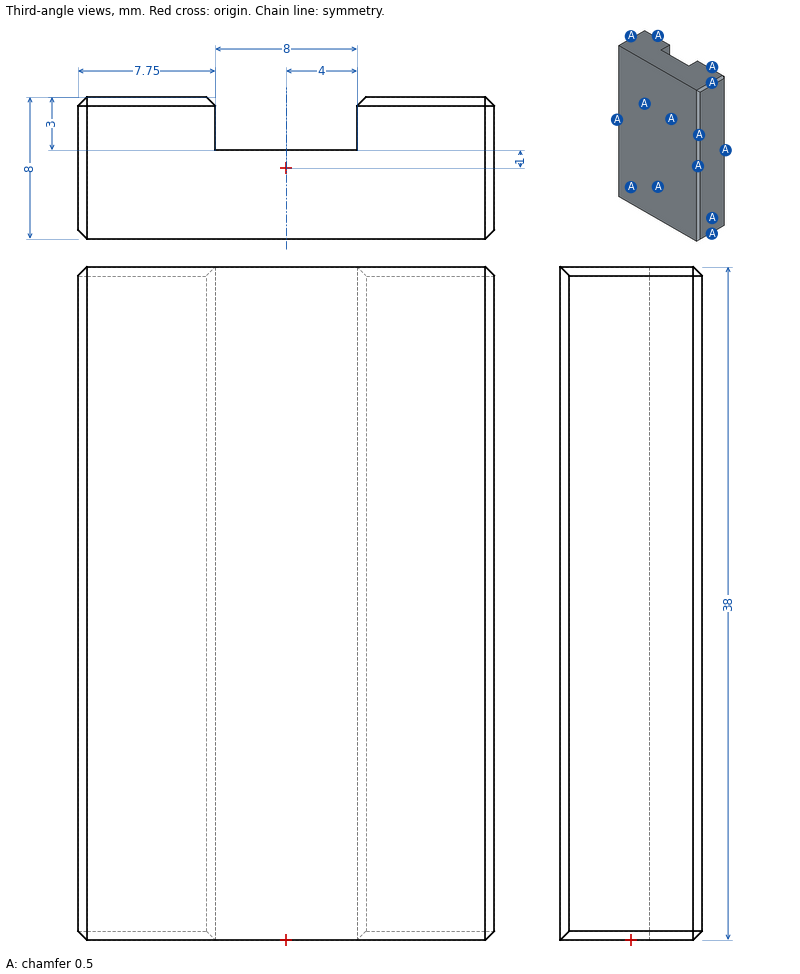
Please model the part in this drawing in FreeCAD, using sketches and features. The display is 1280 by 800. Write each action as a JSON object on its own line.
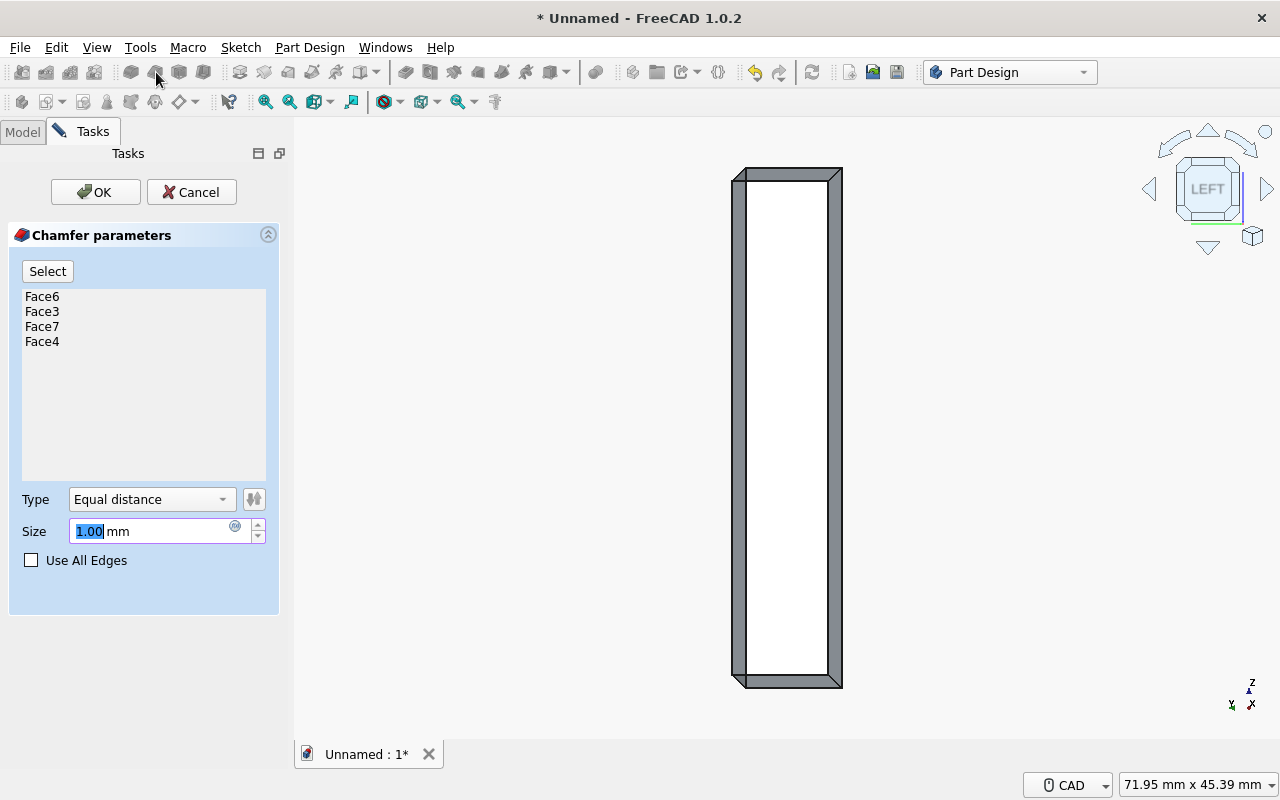
{"action": "type", "text": "0.5"}
{"action": "key", "text": "Tab"}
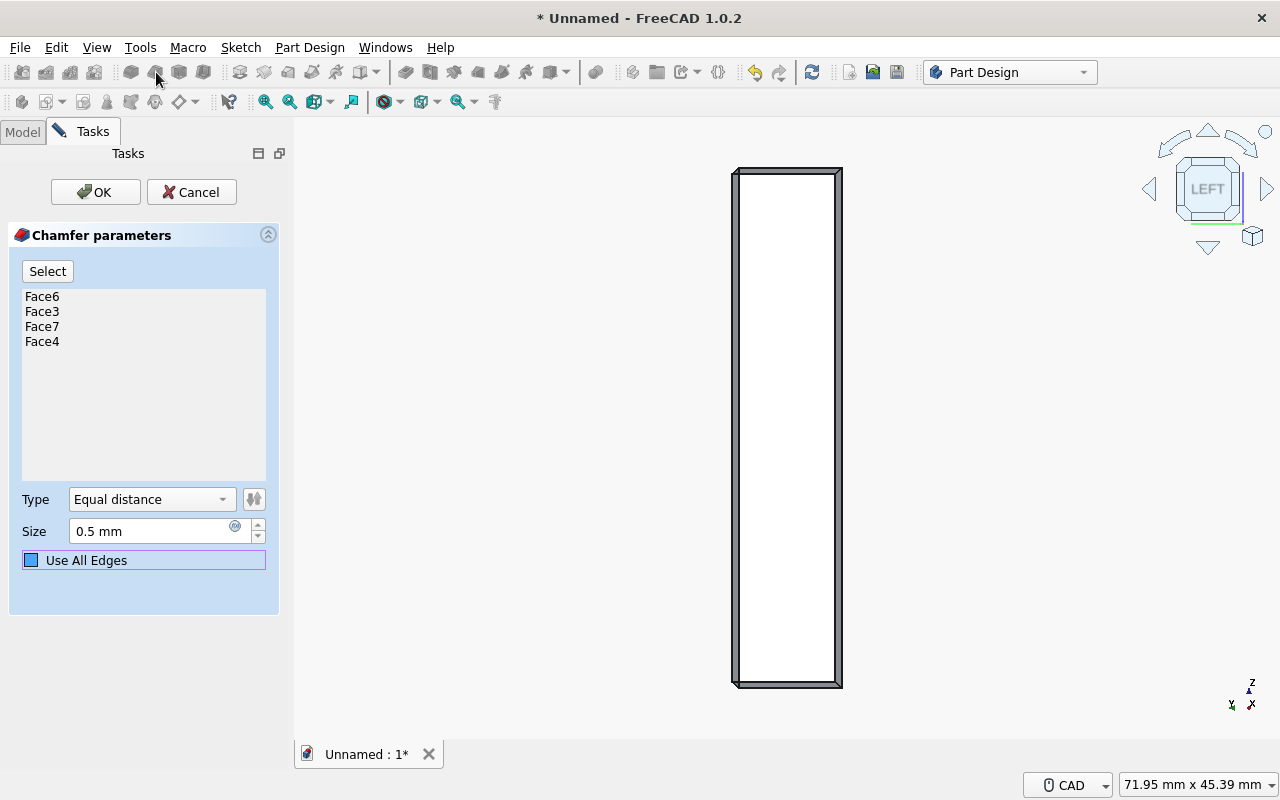
{"action": "left_click", "coordinate": [96, 192]}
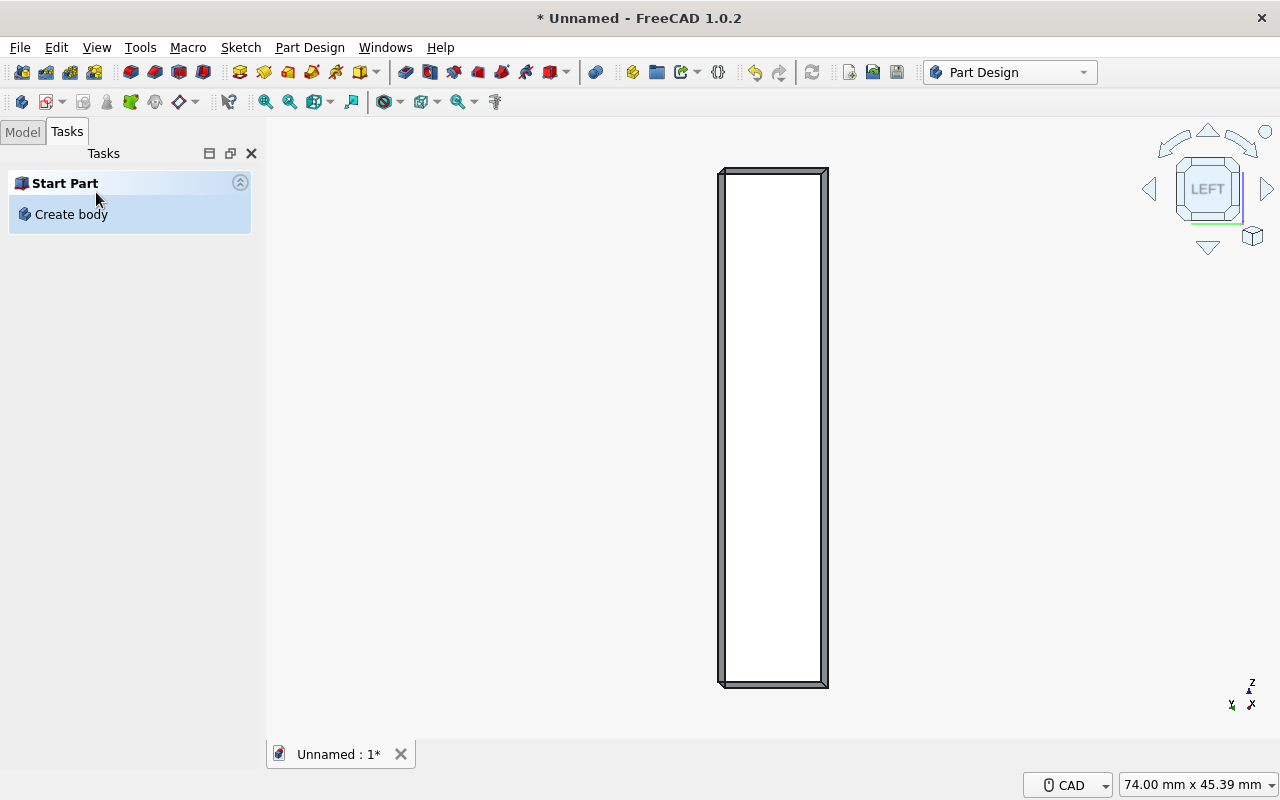
{"action": "key", "text": "0"}